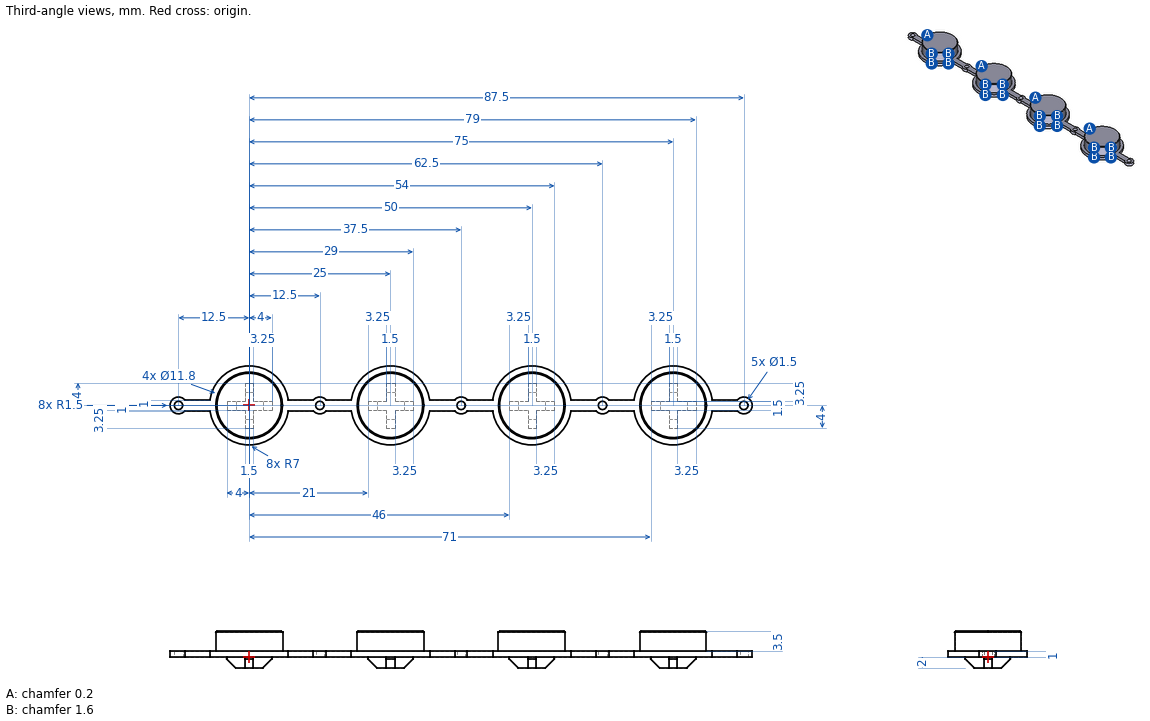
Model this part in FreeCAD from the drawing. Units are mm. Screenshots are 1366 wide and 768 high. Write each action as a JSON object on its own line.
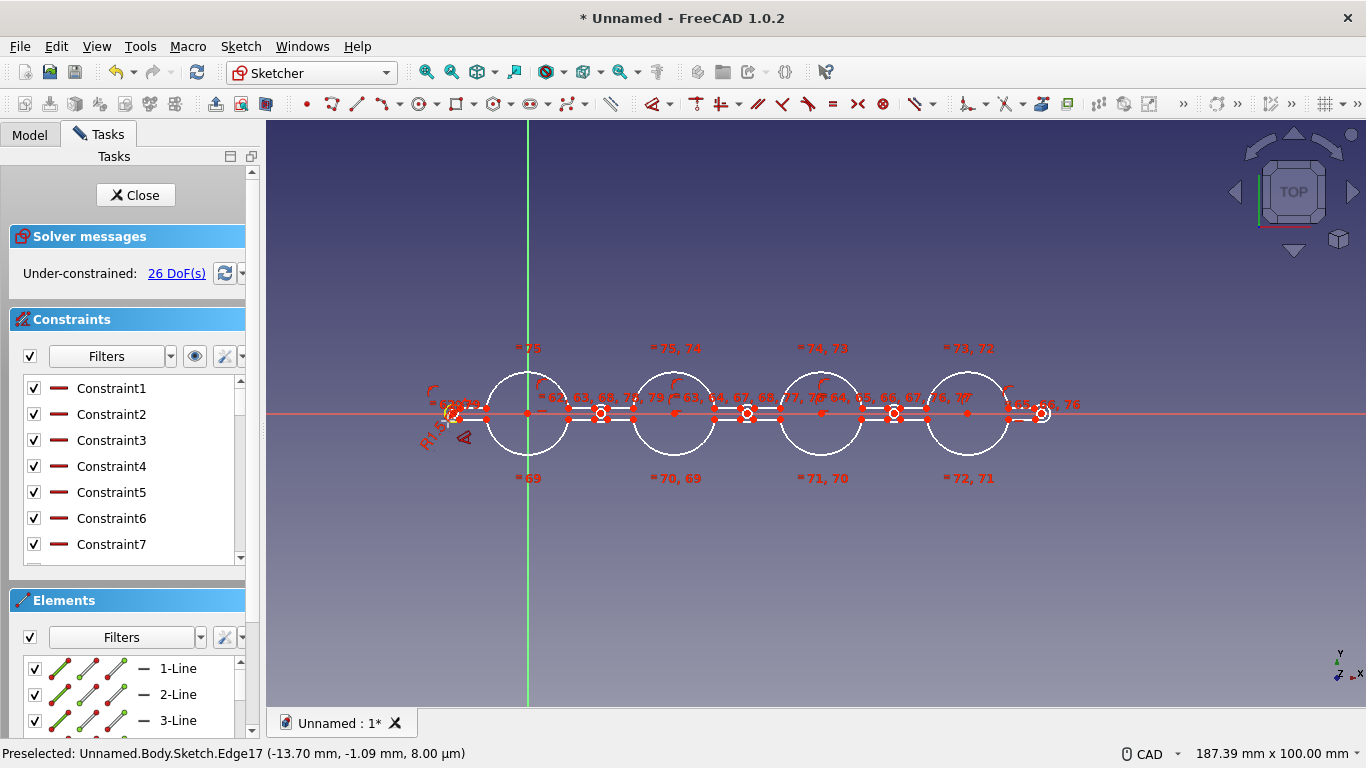
{"action": "left_click", "coordinate": [505, 449]}
{"action": "left_click", "coordinate": [488, 476]}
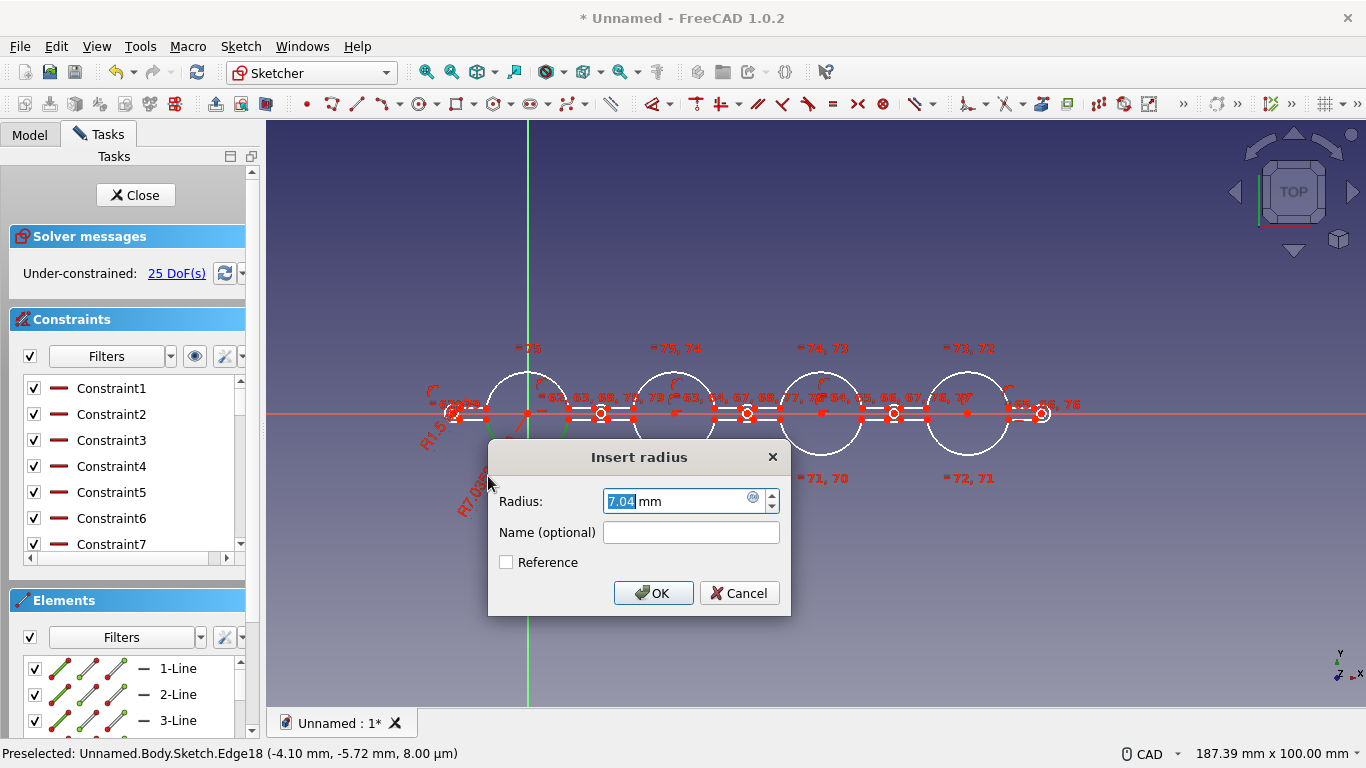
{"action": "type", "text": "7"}
{"action": "key", "text": "Return"}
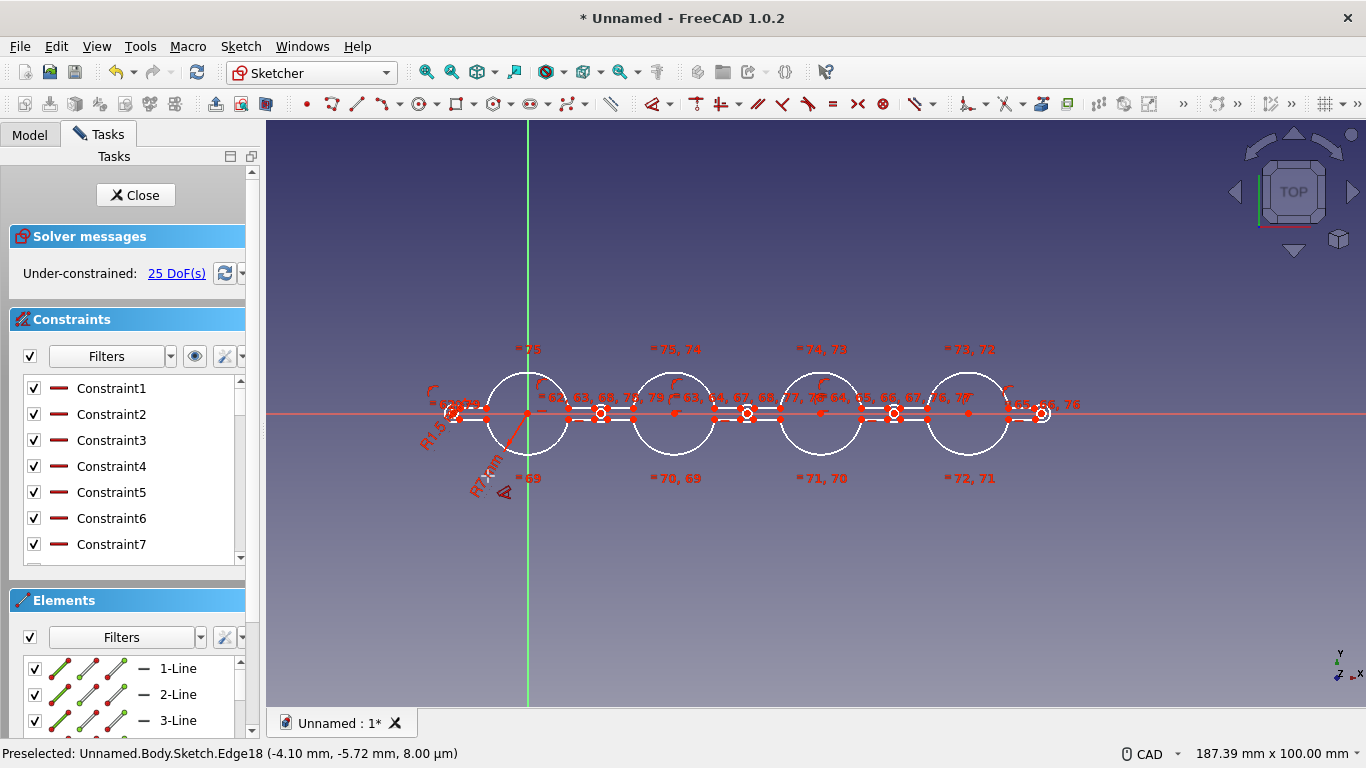
{"action": "scroll", "coordinate": [1037, 414], "scroll_direction": "up", "scroll_amount": 8}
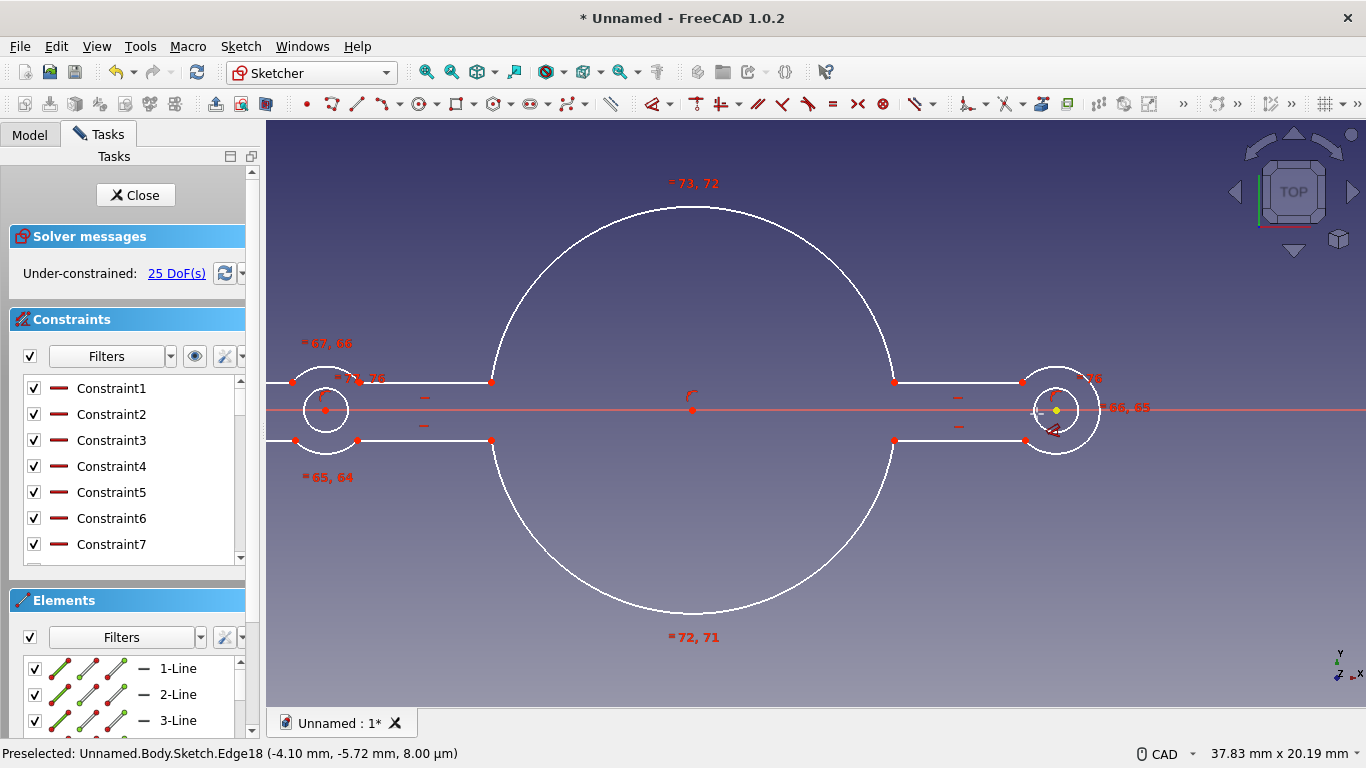
{"action": "left_click", "coordinate": [1034, 410]}
{"action": "left_click", "coordinate": [1015, 345]}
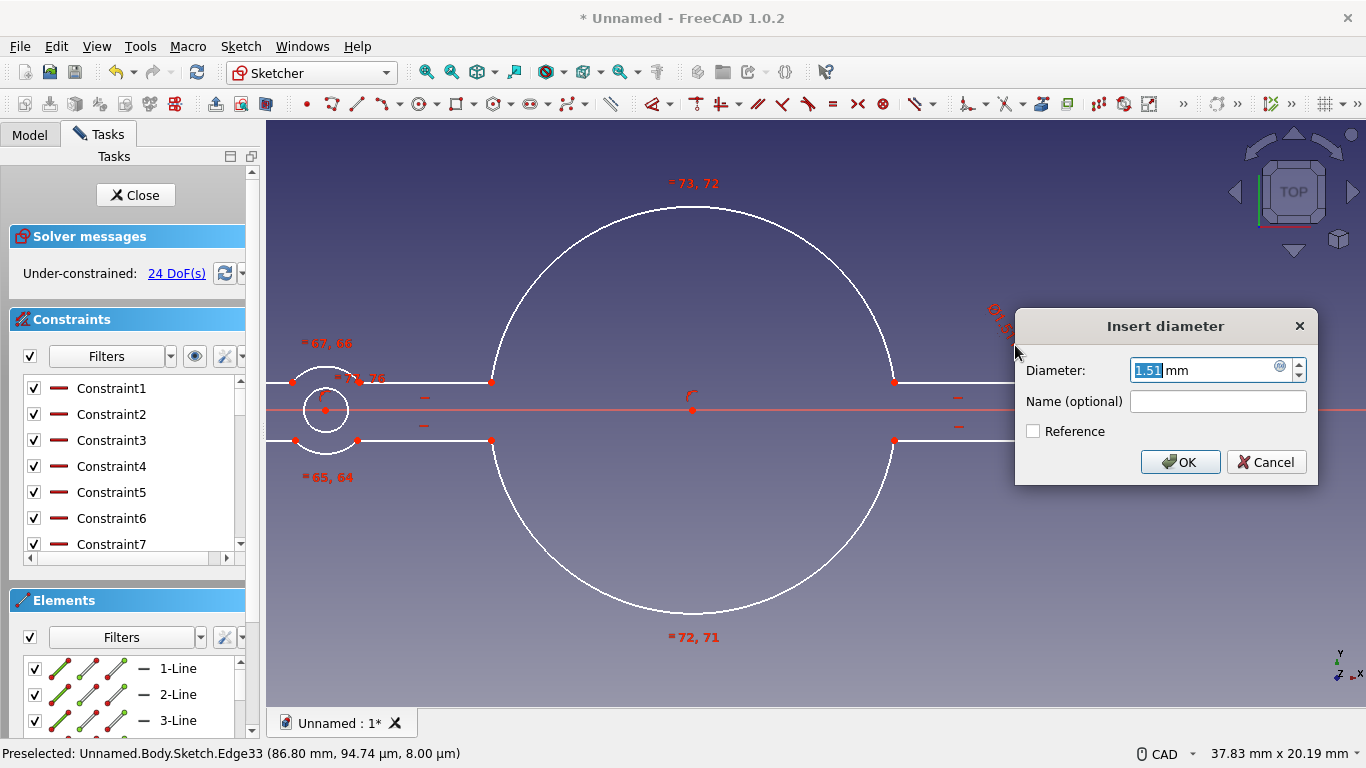
{"action": "type", "text": "1.5"}
{"action": "key", "text": "Return"}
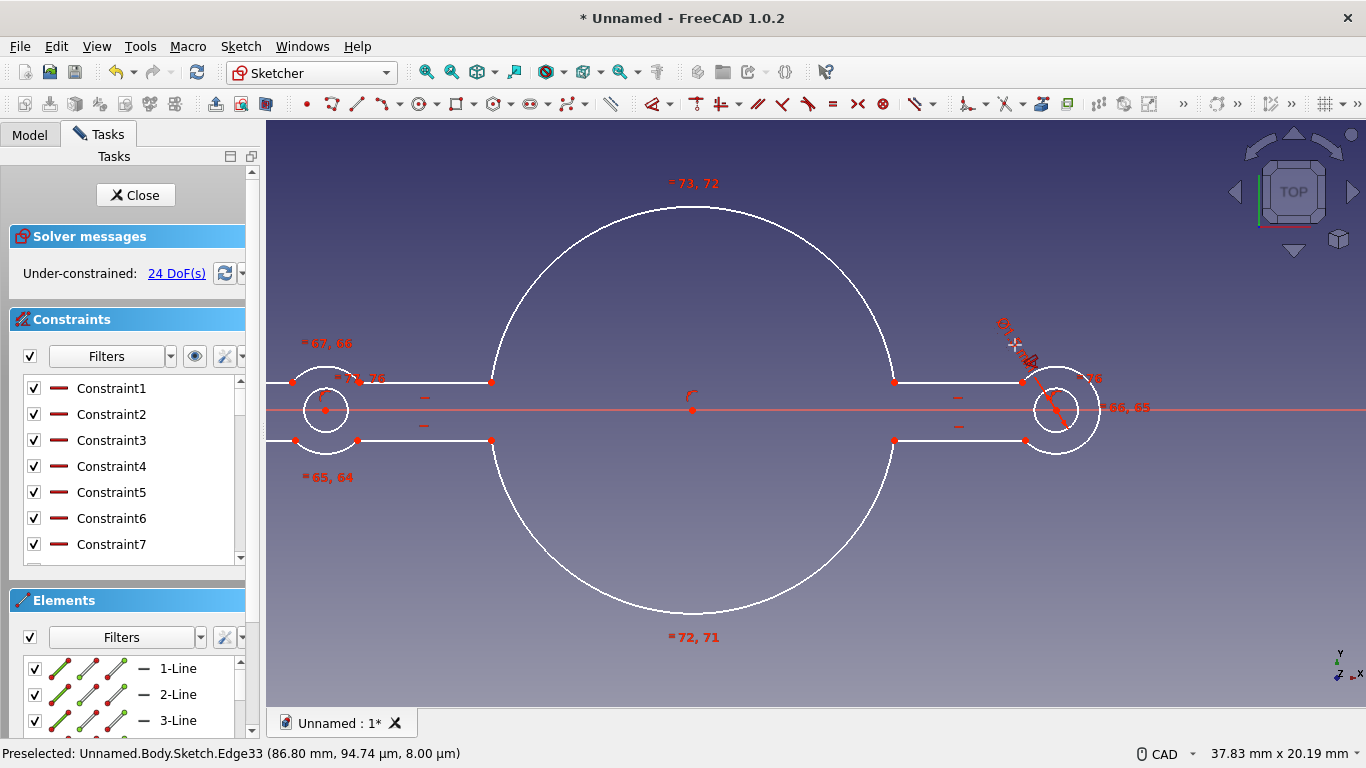
{"action": "scroll", "coordinate": [1038, 414], "scroll_direction": "down", "scroll_amount": 8}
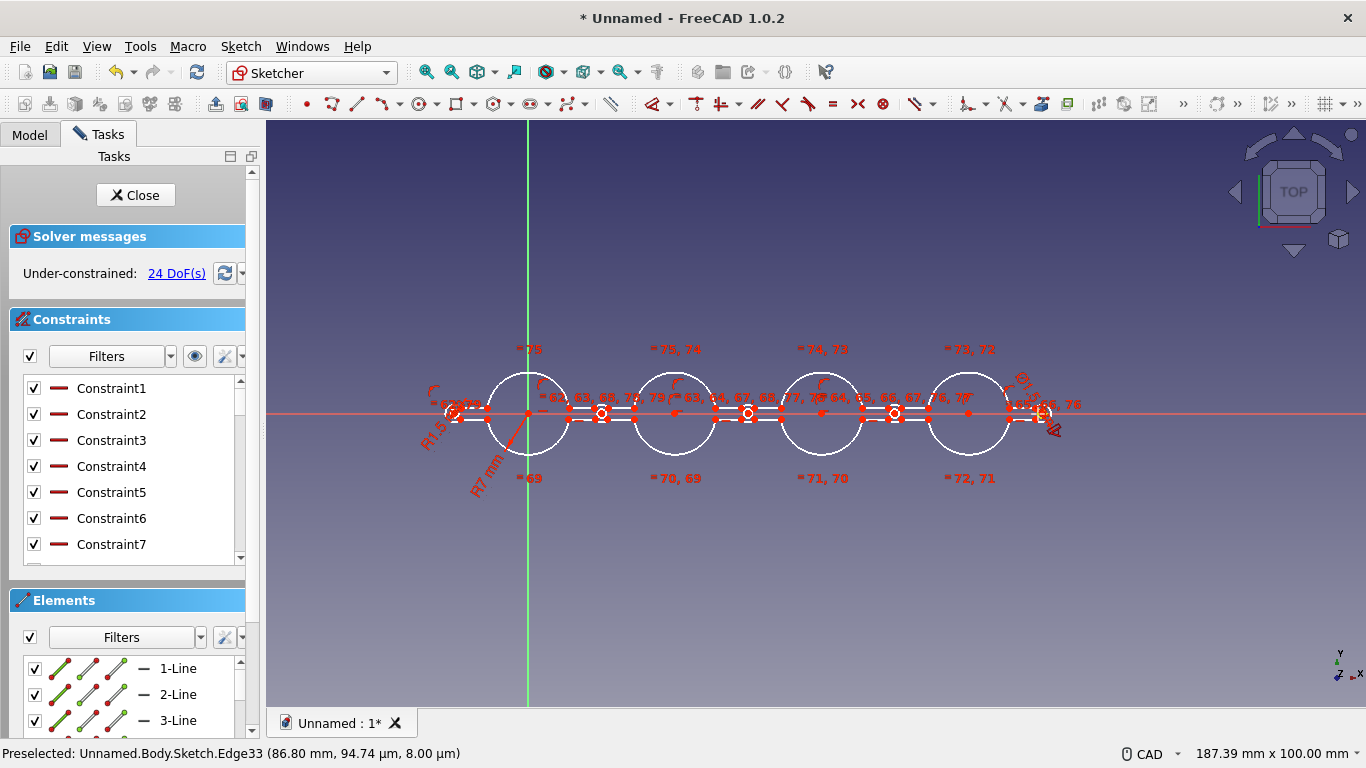
{"action": "scroll", "coordinate": [488, 408], "scroll_direction": "up", "scroll_amount": 10}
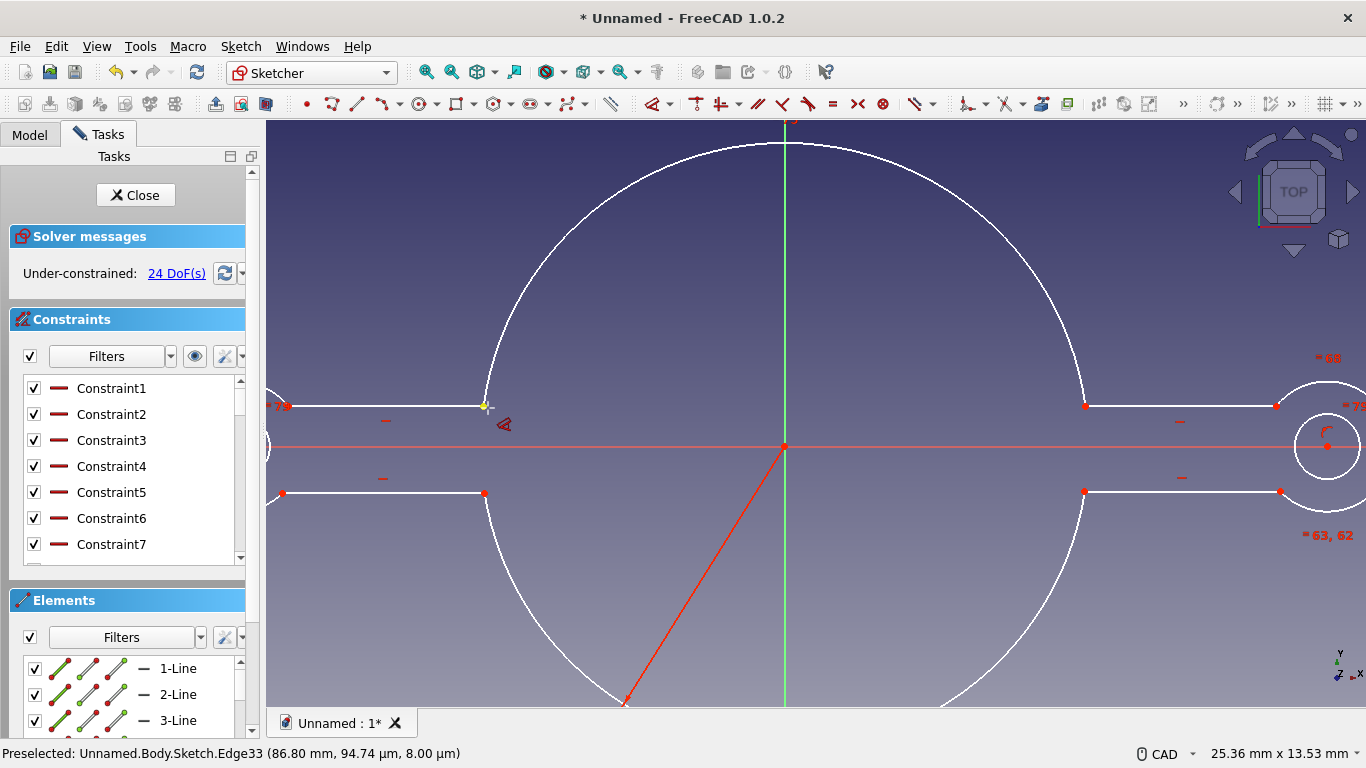
{"action": "left_click", "coordinate": [484, 406]}
{"action": "left_click", "coordinate": [450, 426]}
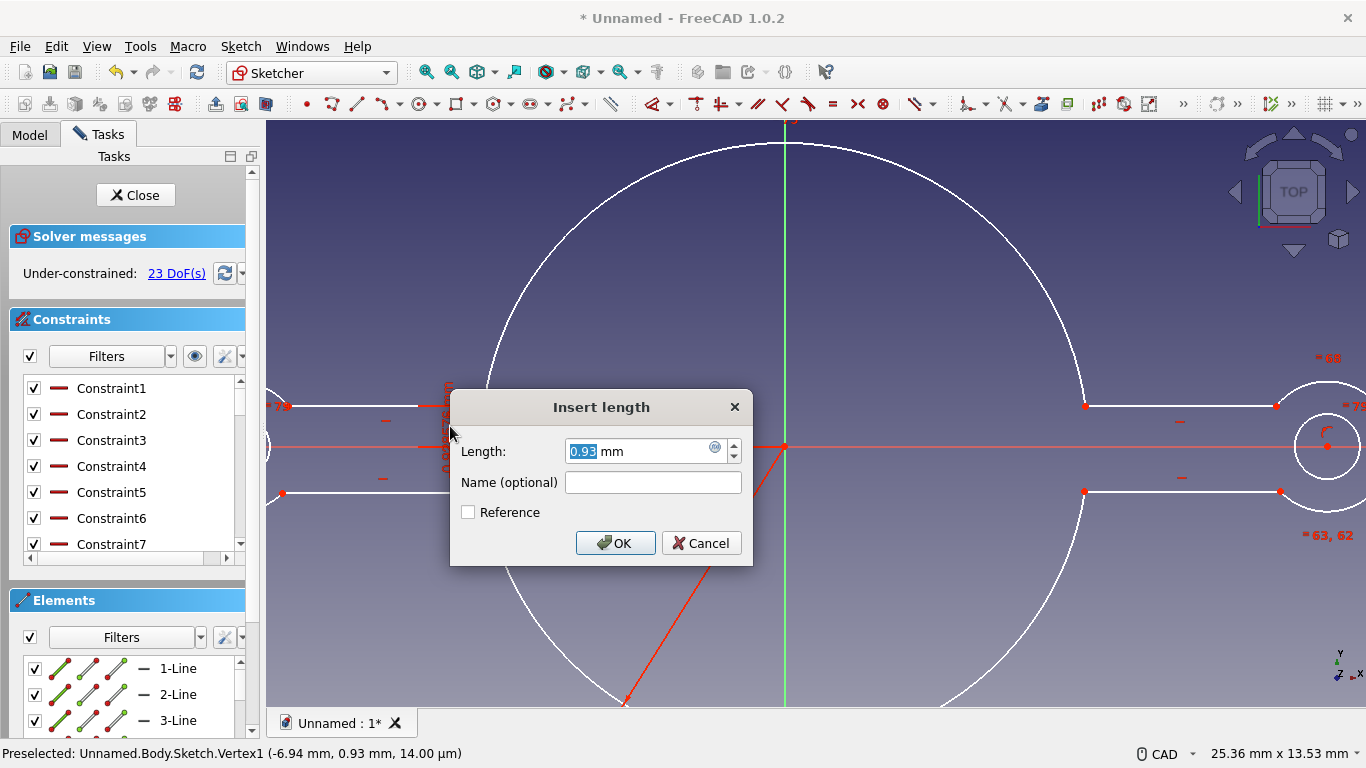
{"action": "type", "text": "1"}
{"action": "key", "text": "Return"}